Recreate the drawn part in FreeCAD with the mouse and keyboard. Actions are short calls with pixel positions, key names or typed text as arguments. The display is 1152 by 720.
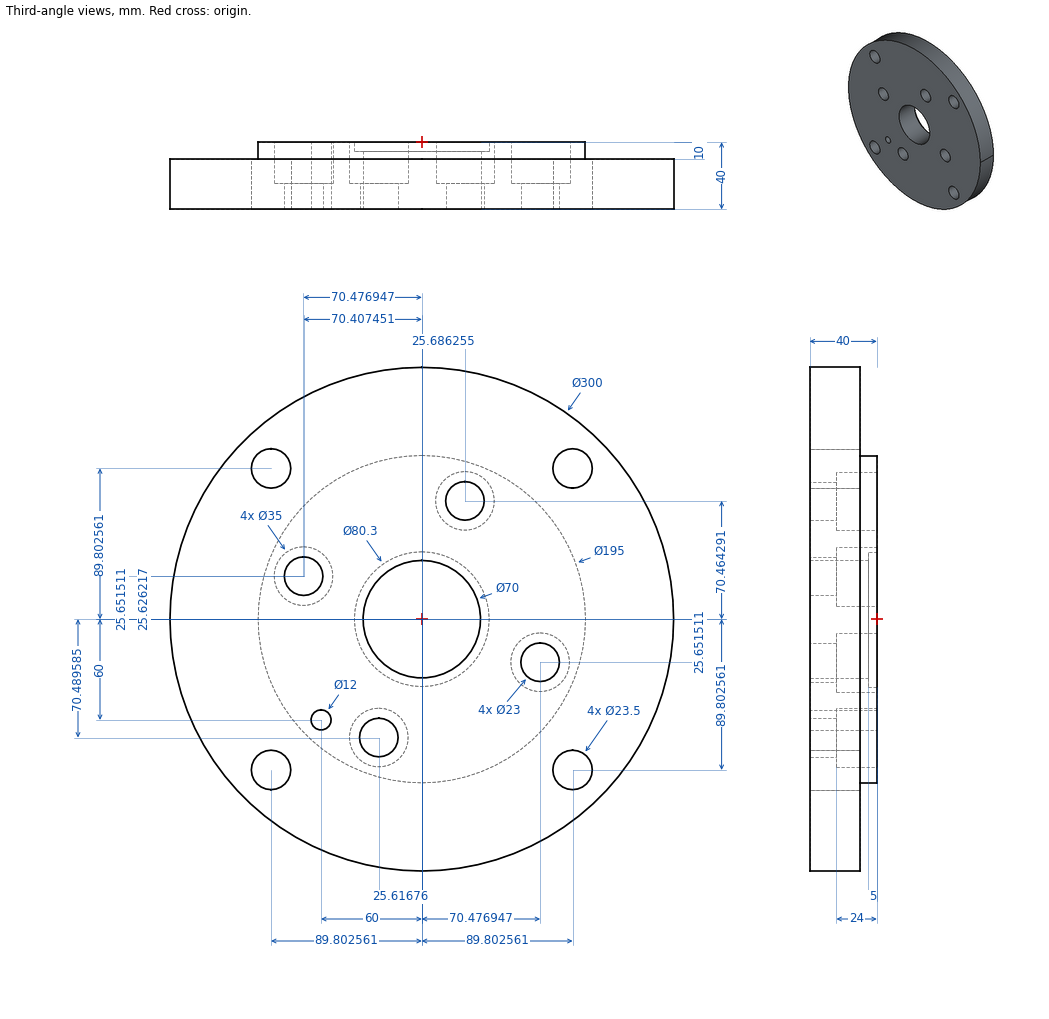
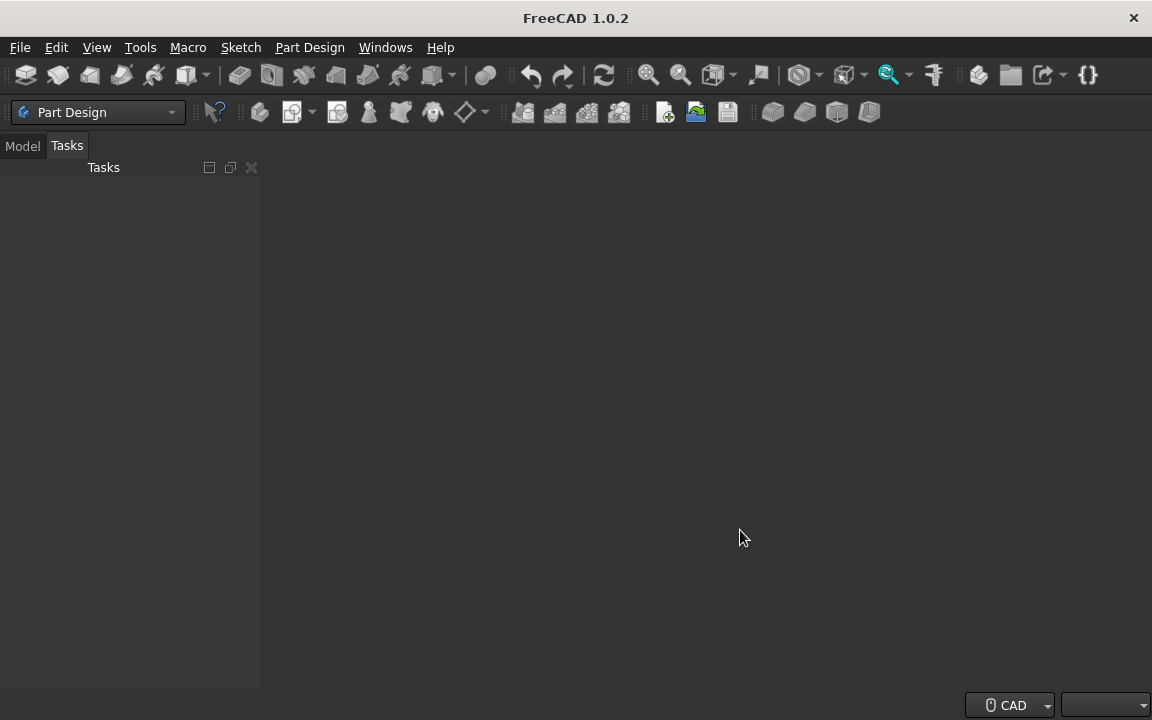
click(664, 112)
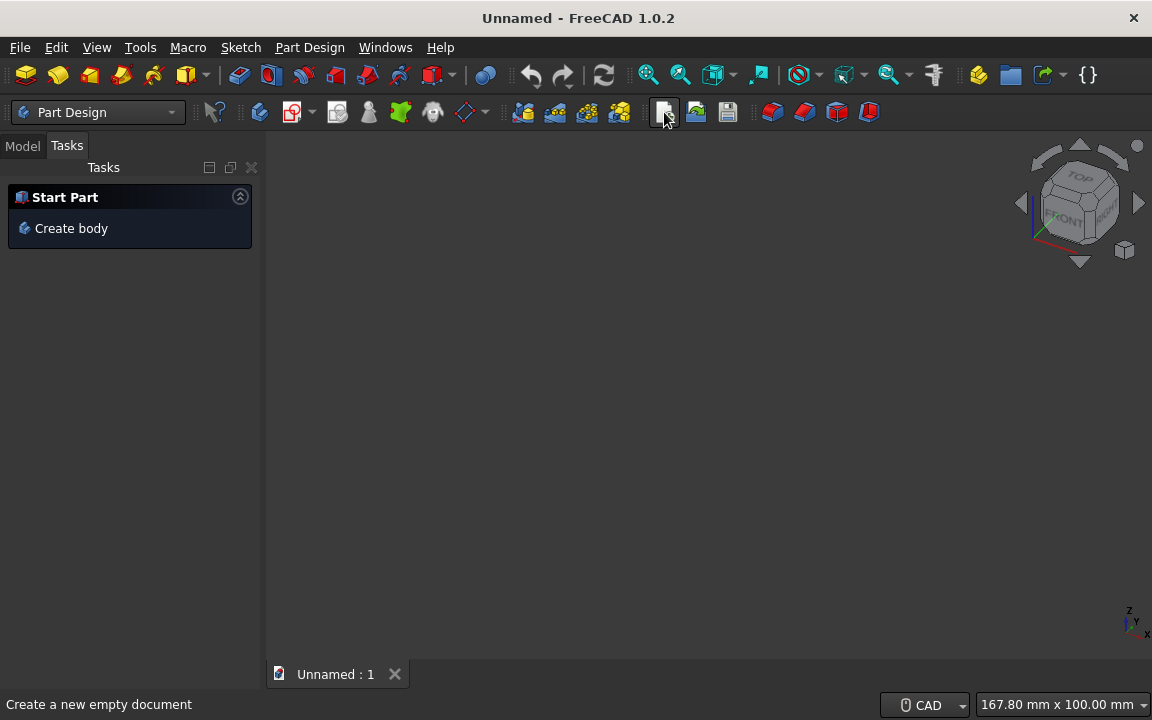
click(292, 112)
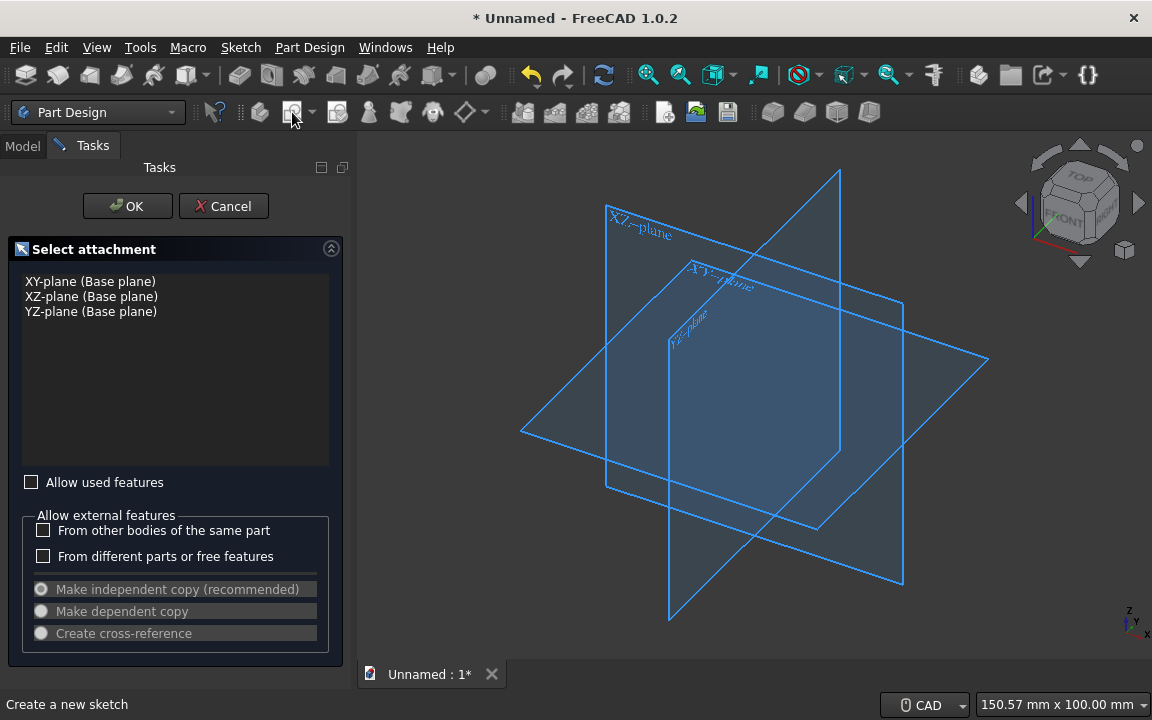
click(82, 296)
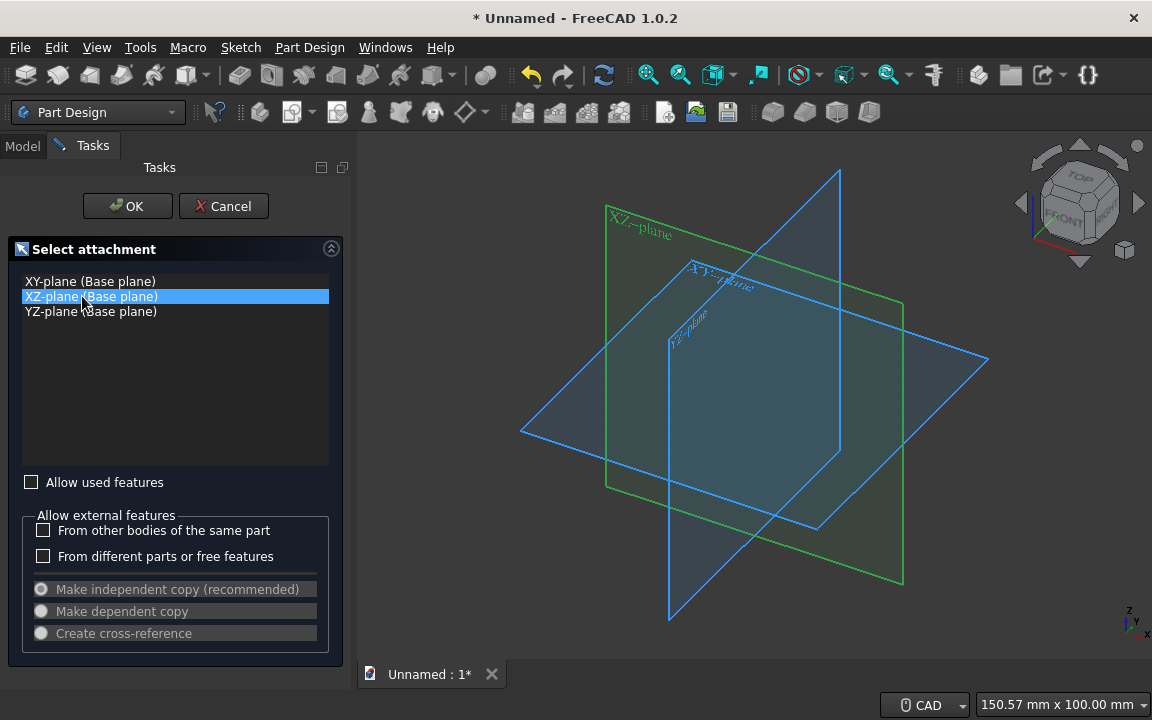
click(128, 206)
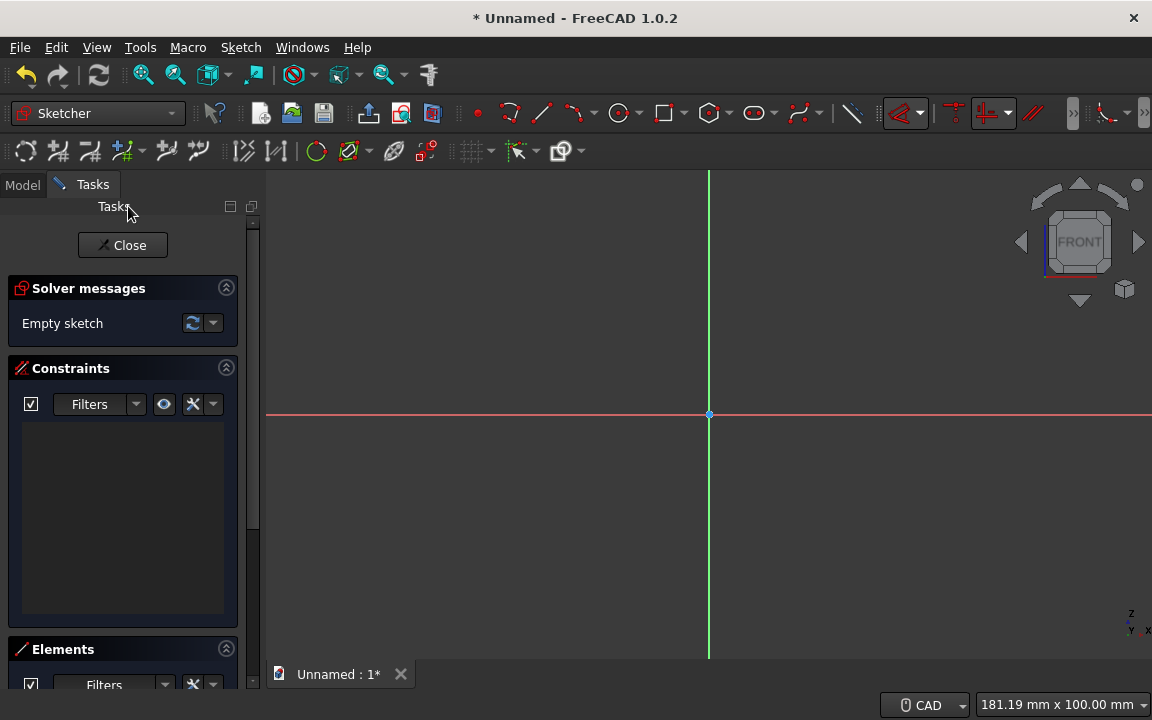
scroll(623, 414, down, 8)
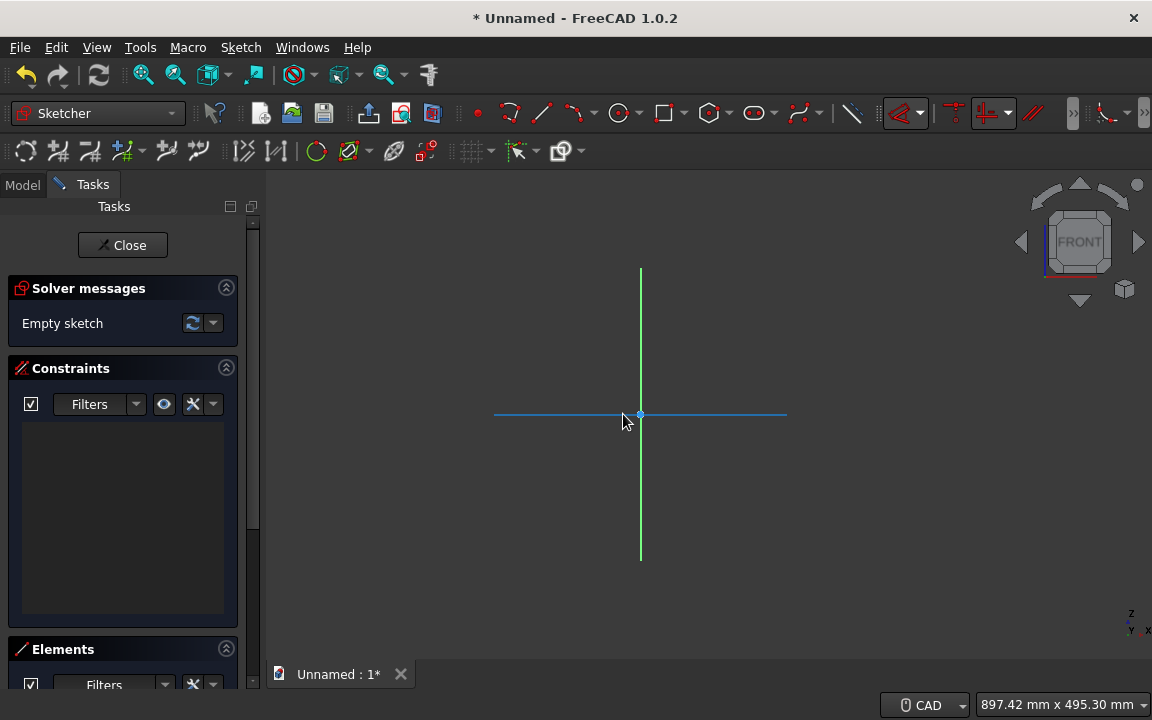
click(620, 114)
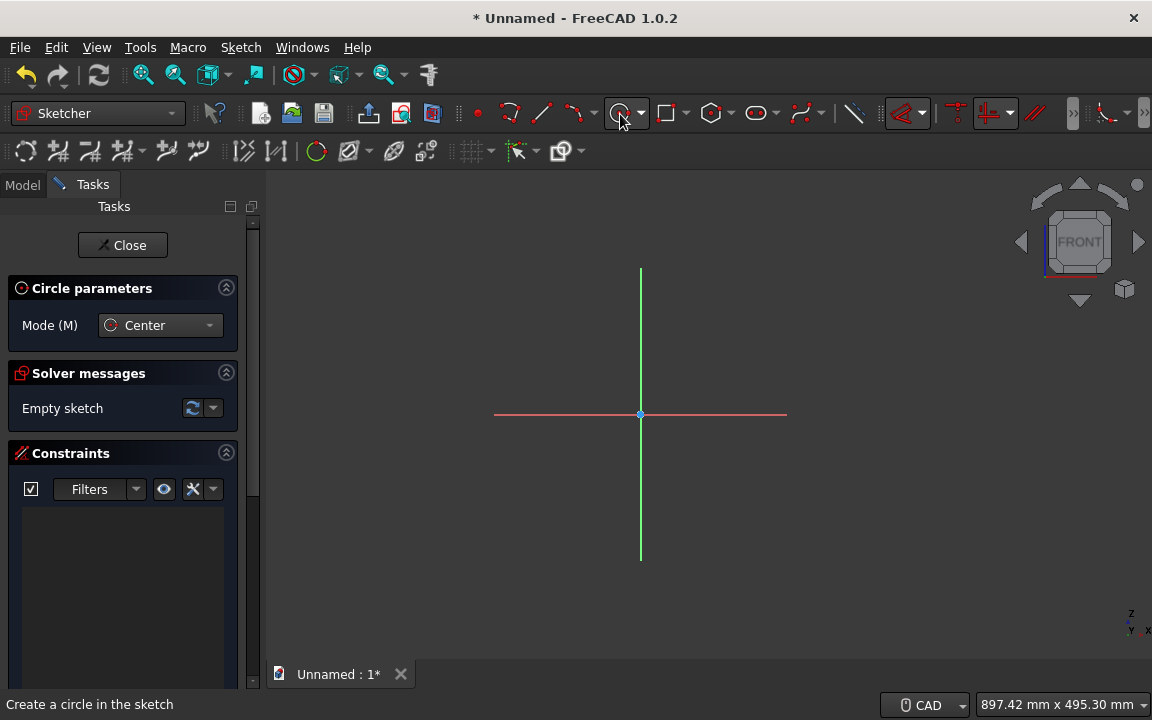
click(641, 414)
move(745, 310)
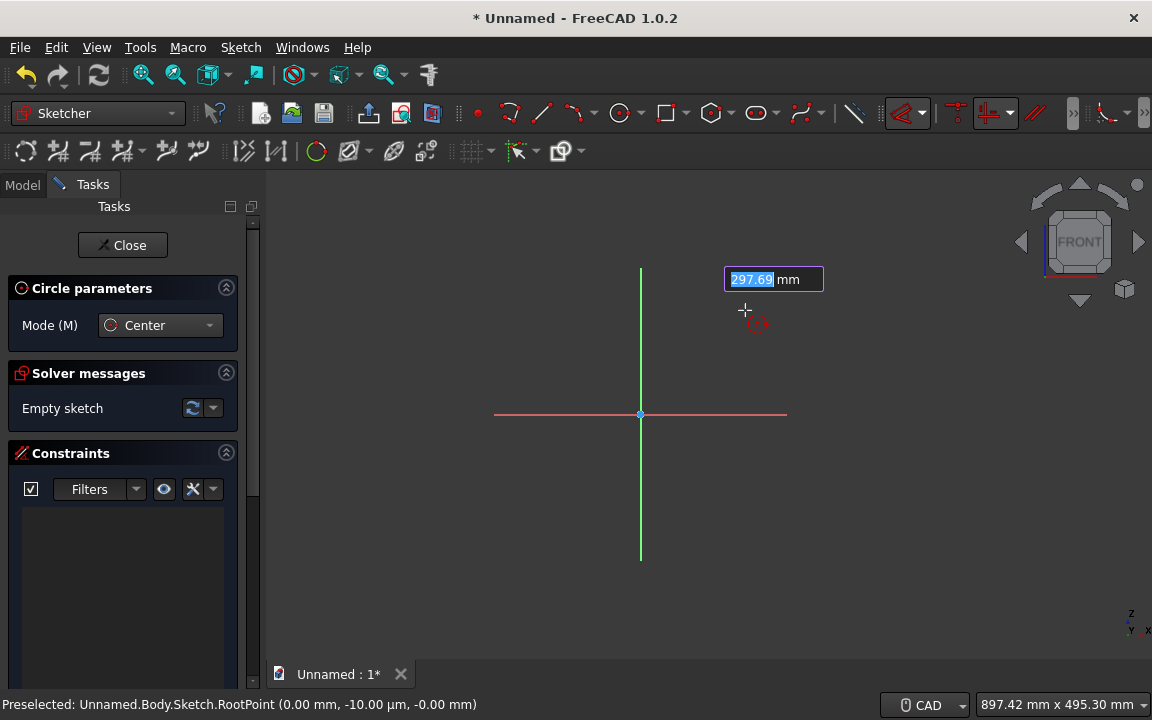
text(300)
key(Return)
key(Escape)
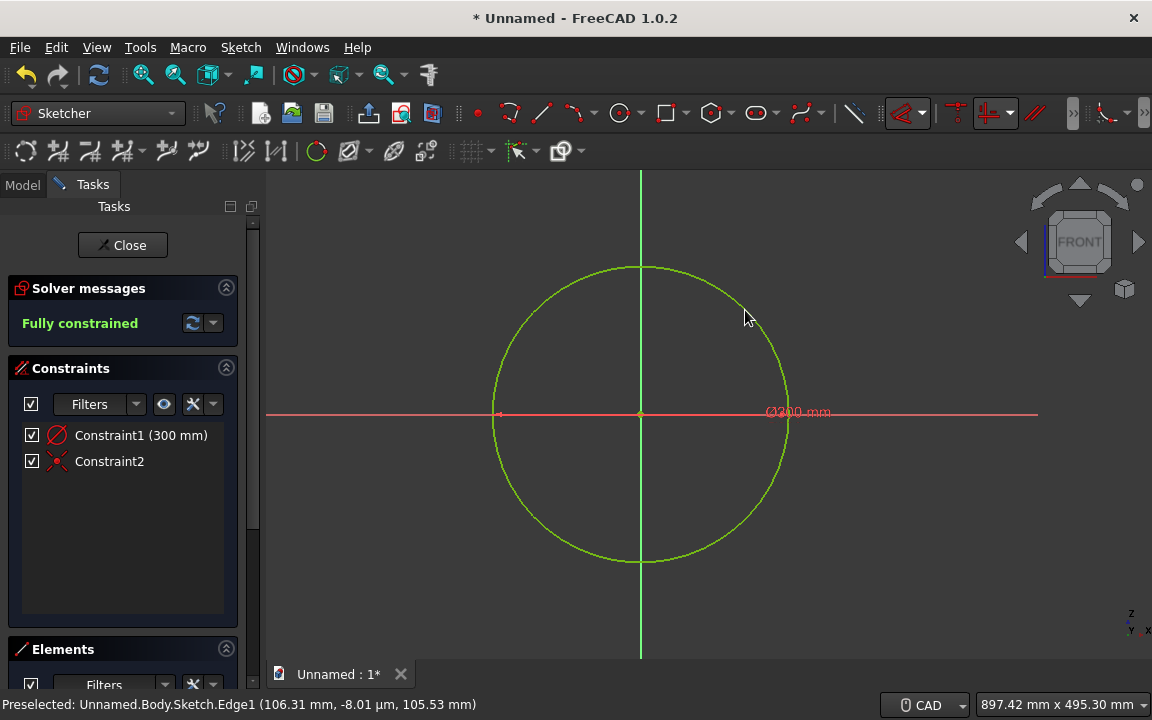
click(123, 245)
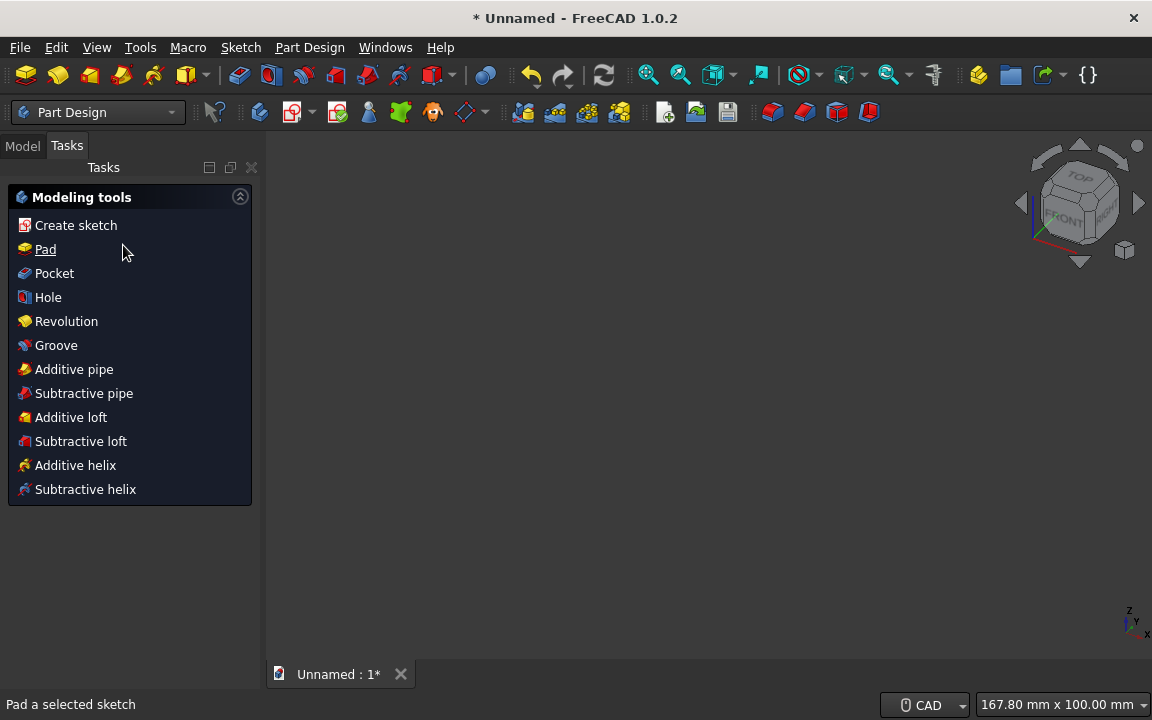
click(26, 76)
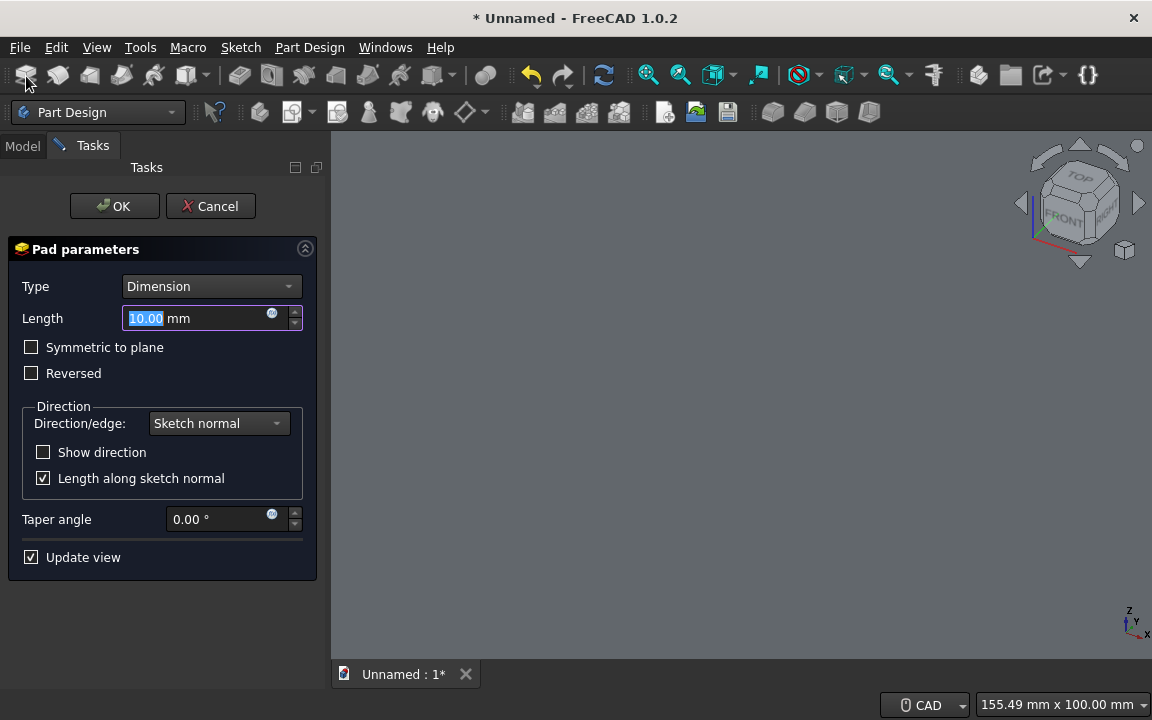
text(40)
key(Tab)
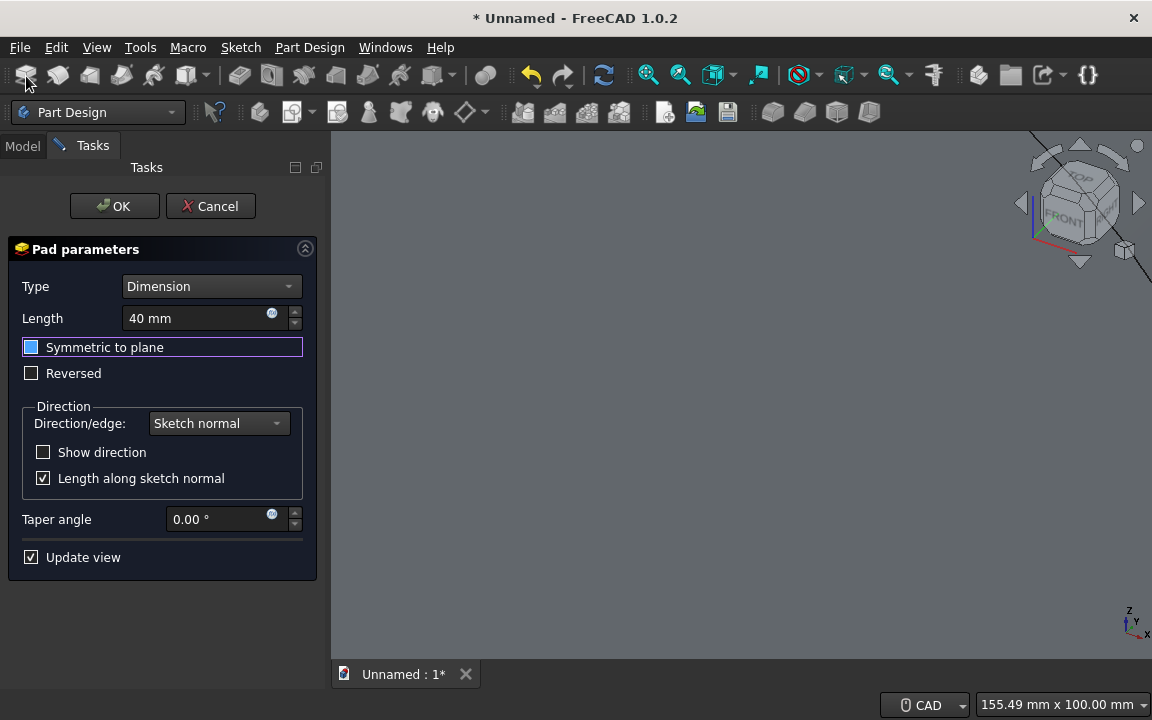
click(115, 206)